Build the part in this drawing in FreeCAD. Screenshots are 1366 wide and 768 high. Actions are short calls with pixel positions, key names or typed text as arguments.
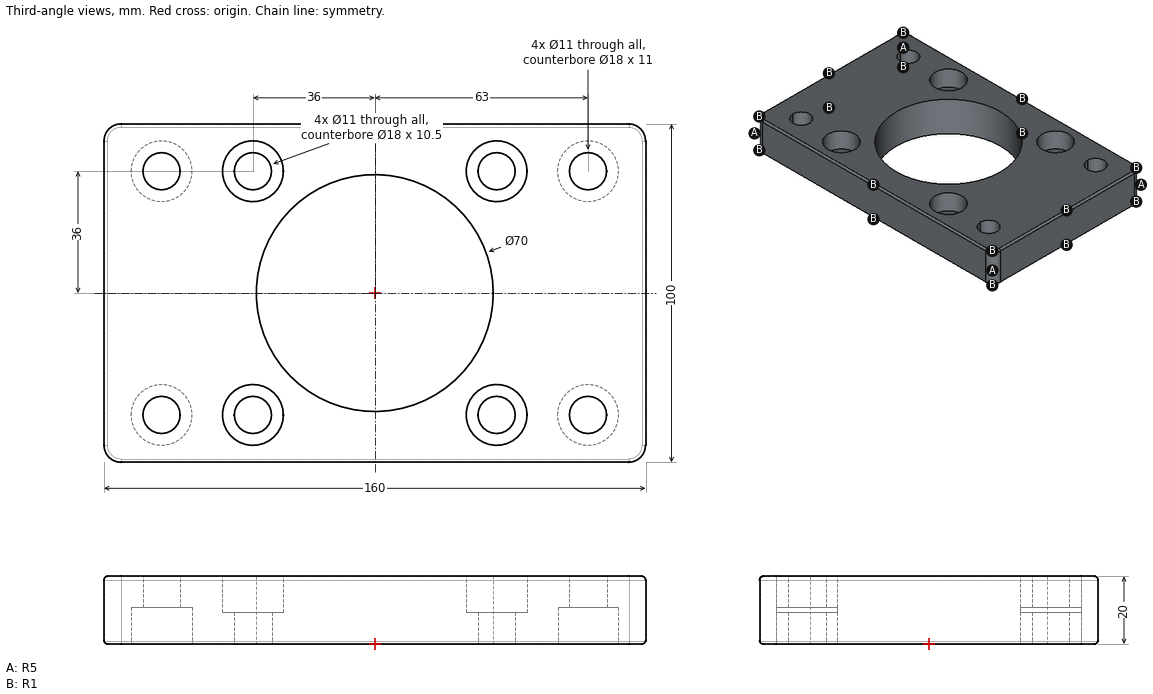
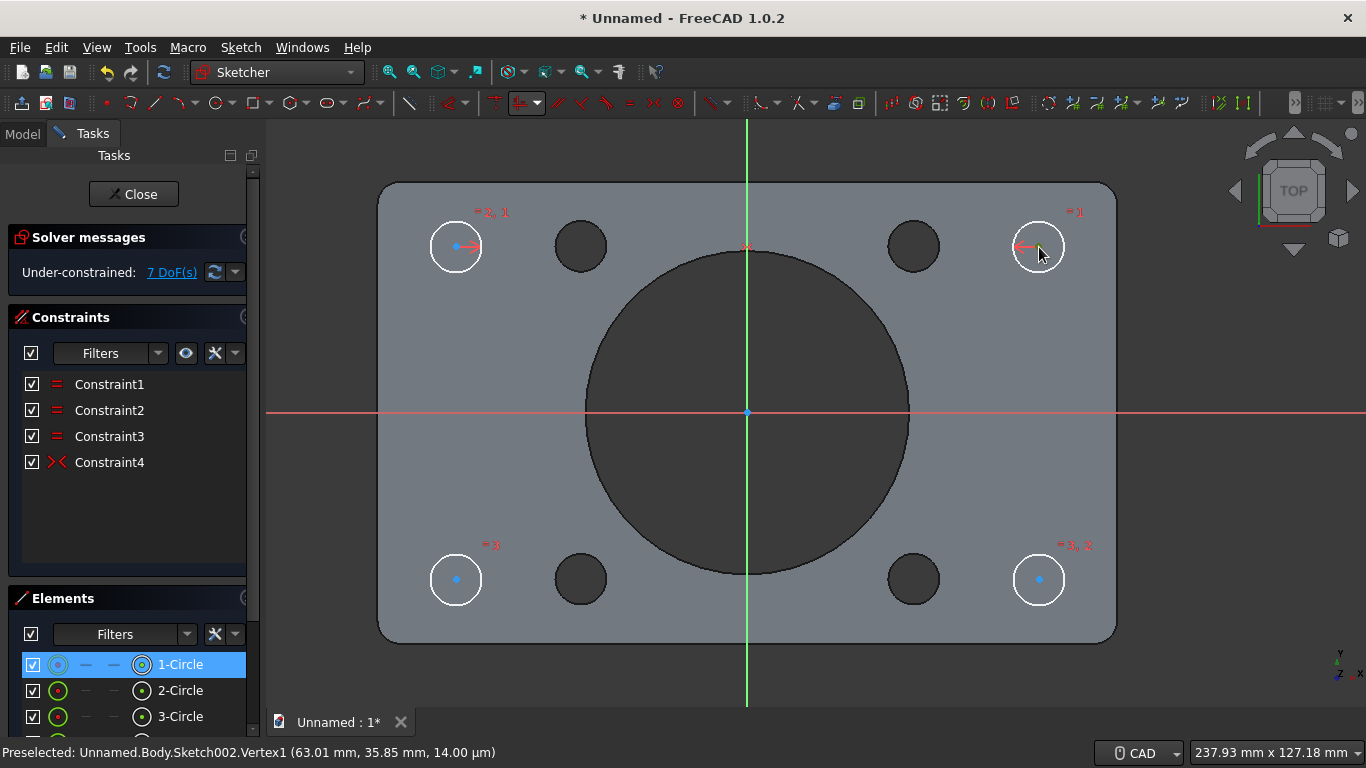
click(1039, 580)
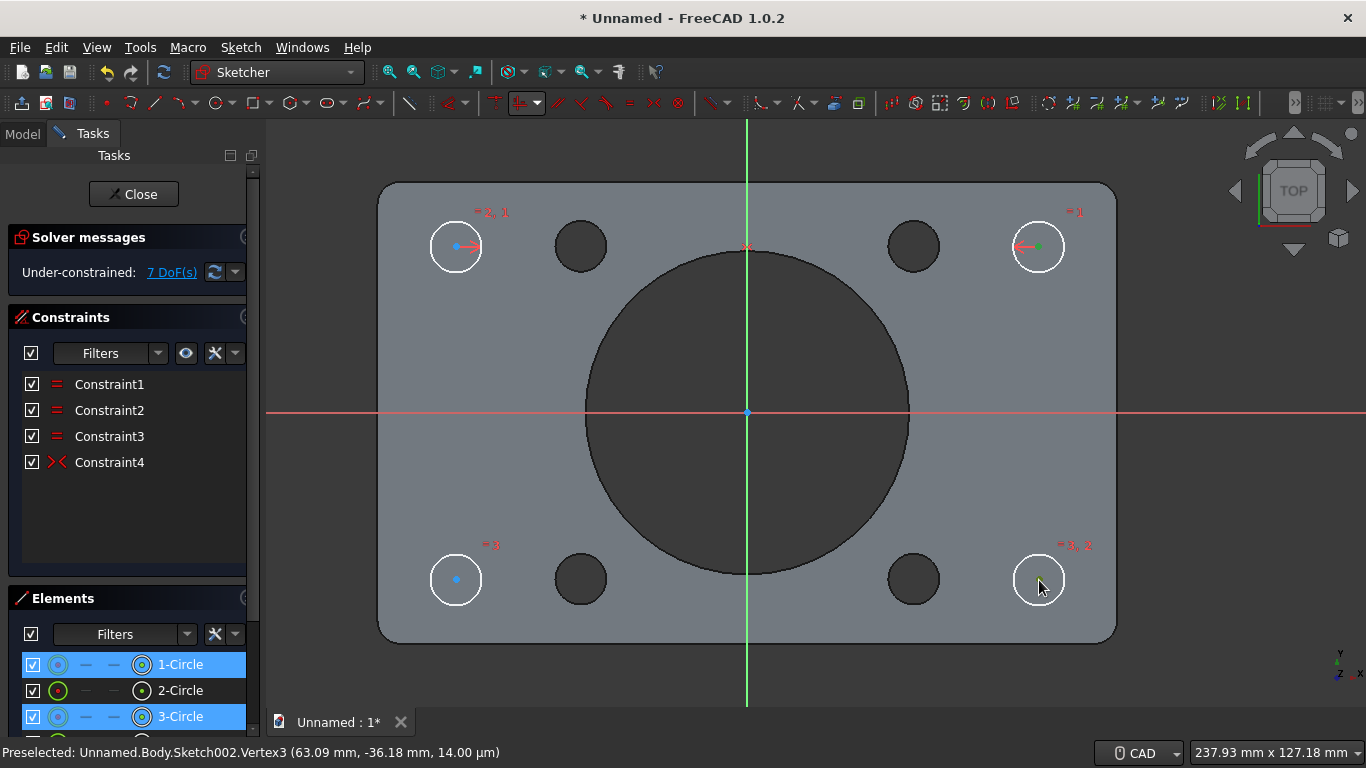
click(359, 413)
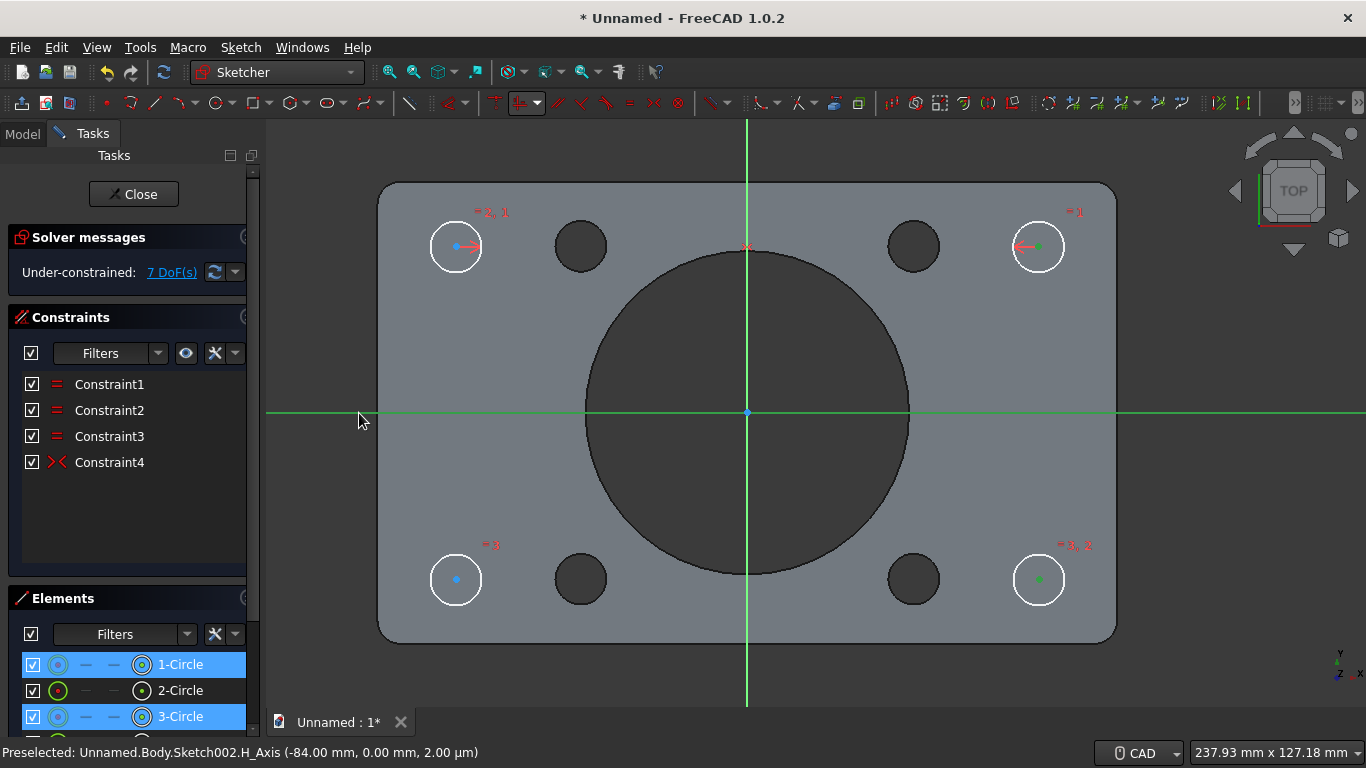
click(654, 104)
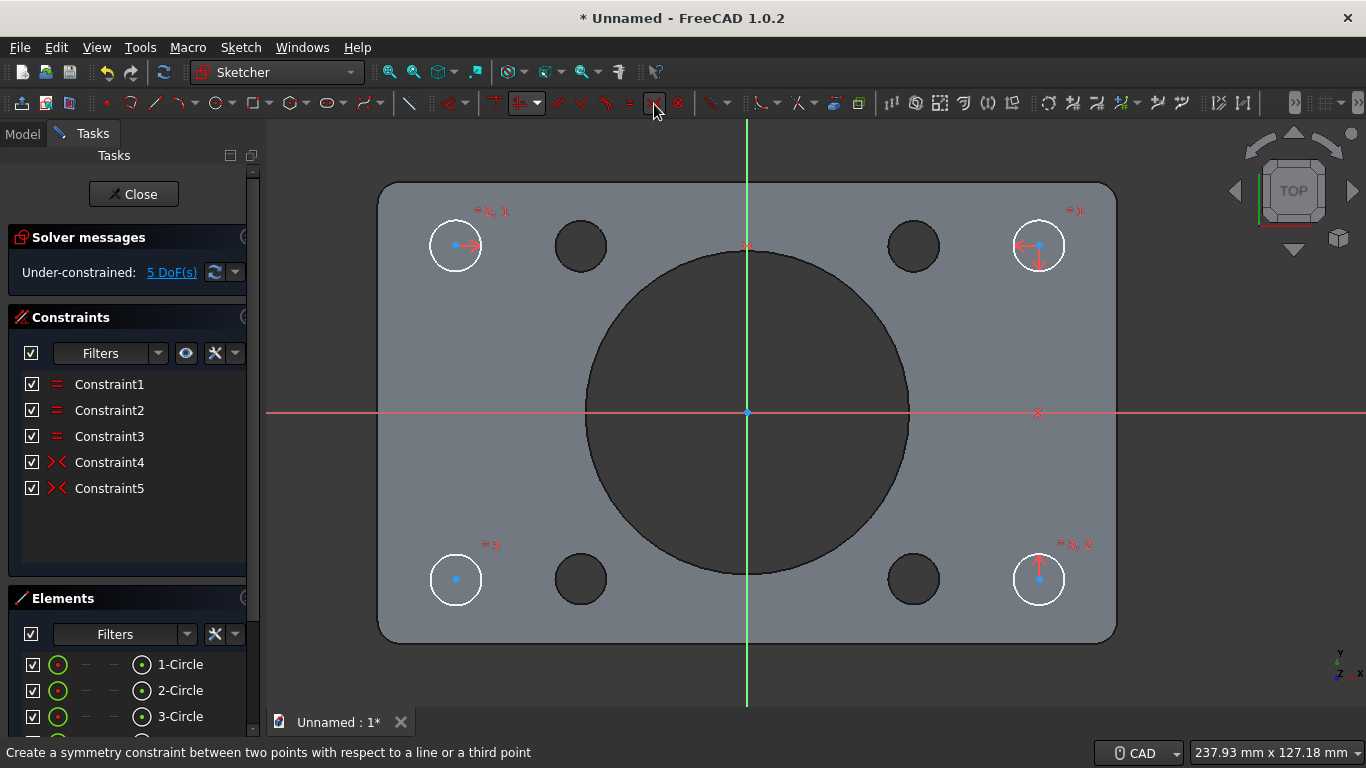
click(456, 246)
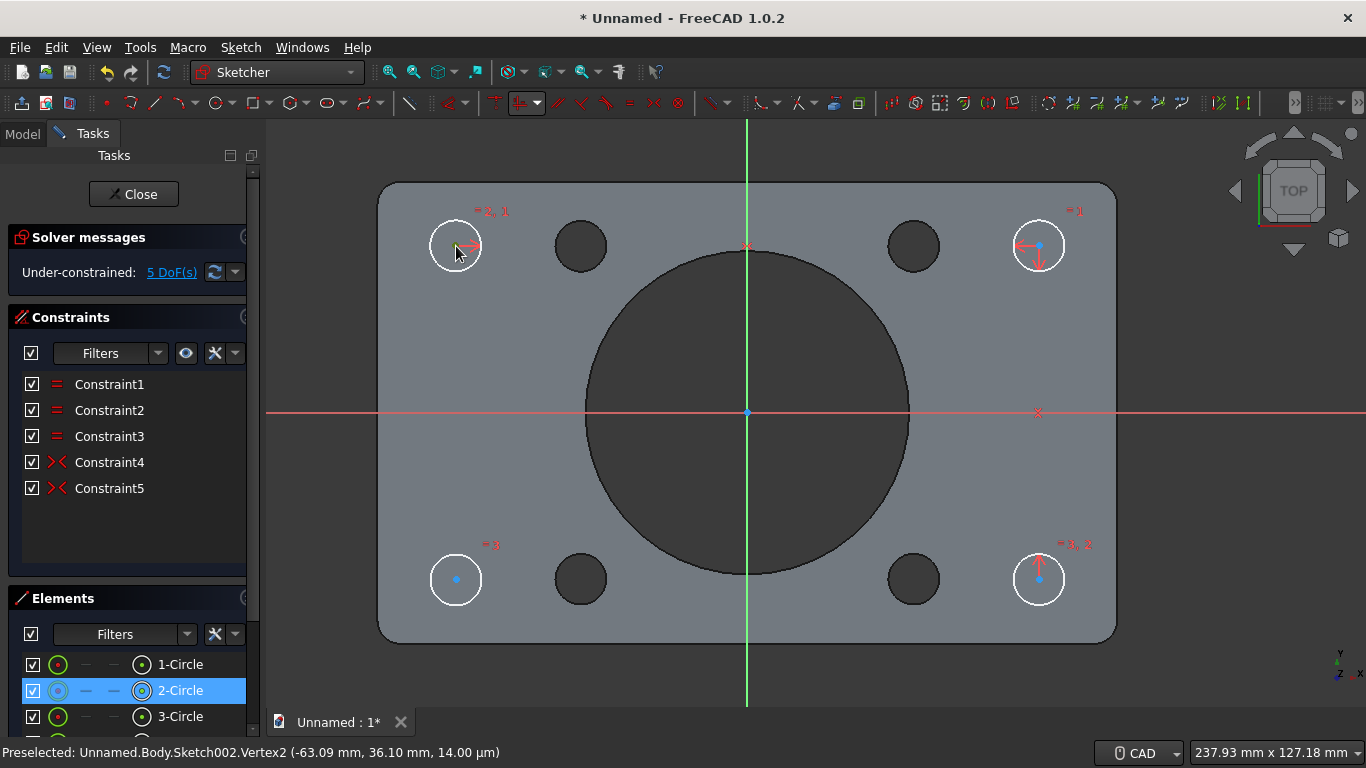
click(456, 580)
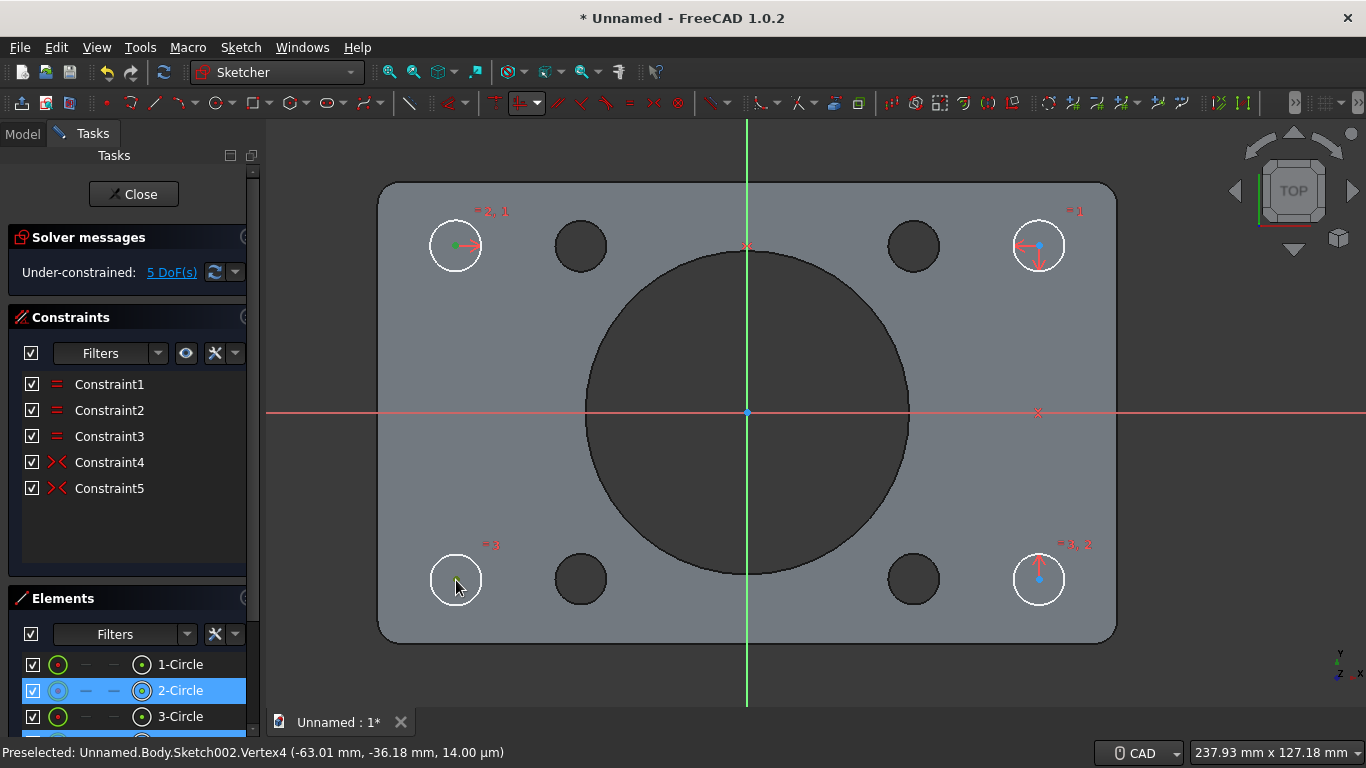
click(359, 413)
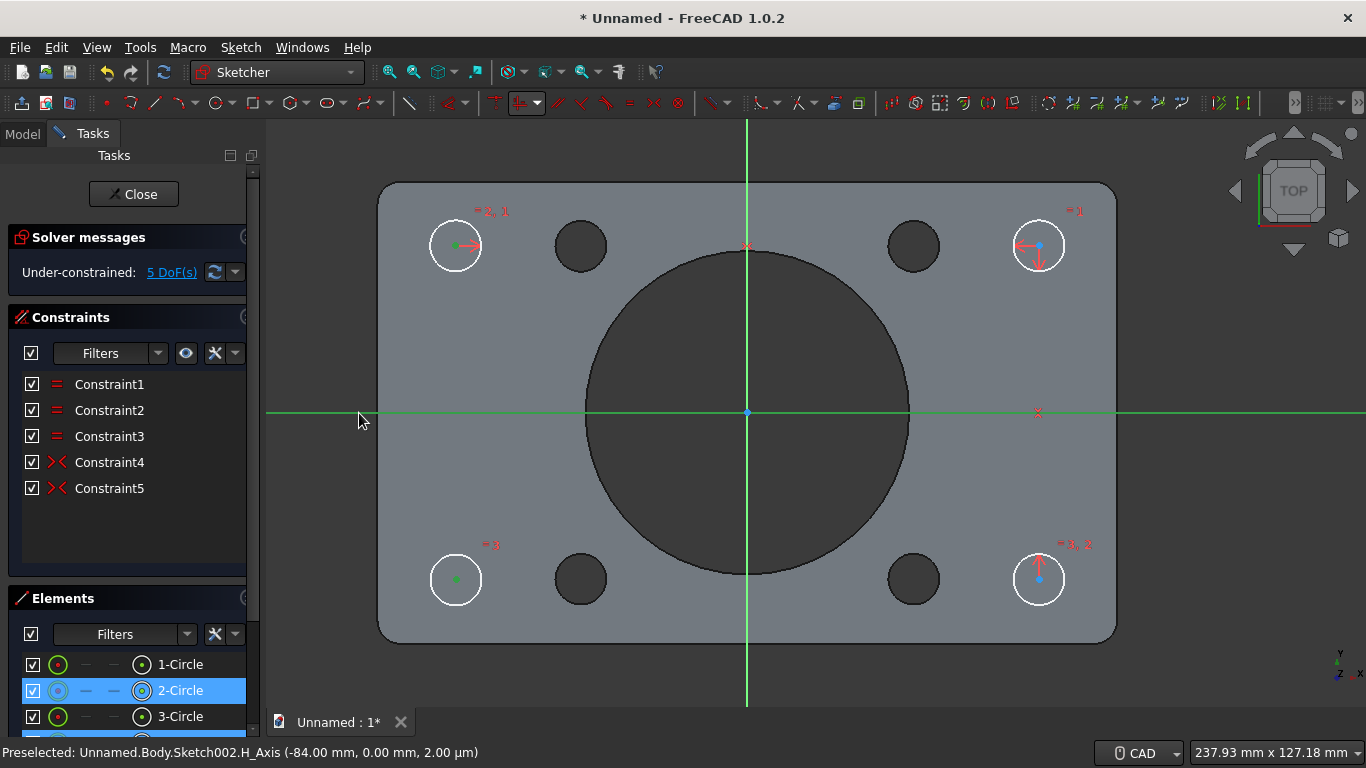
click(654, 104)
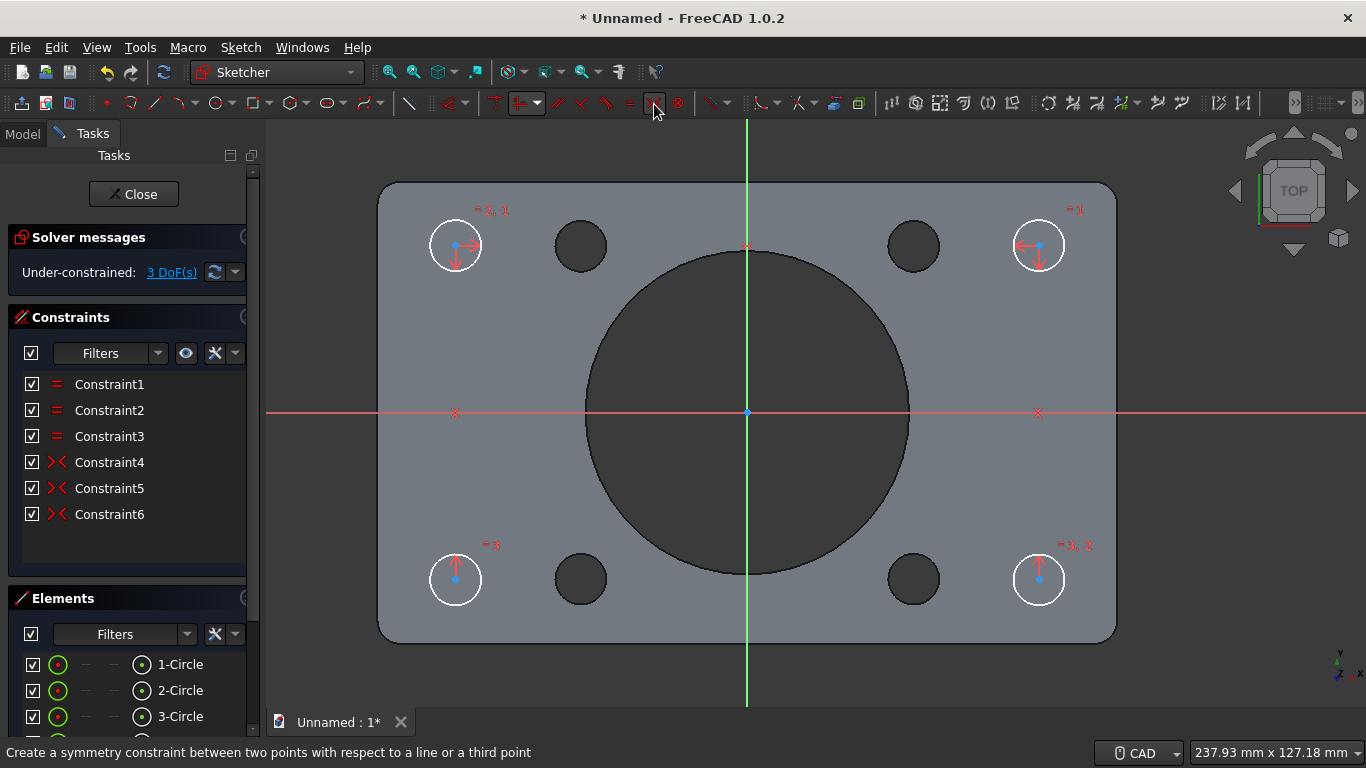
click(448, 104)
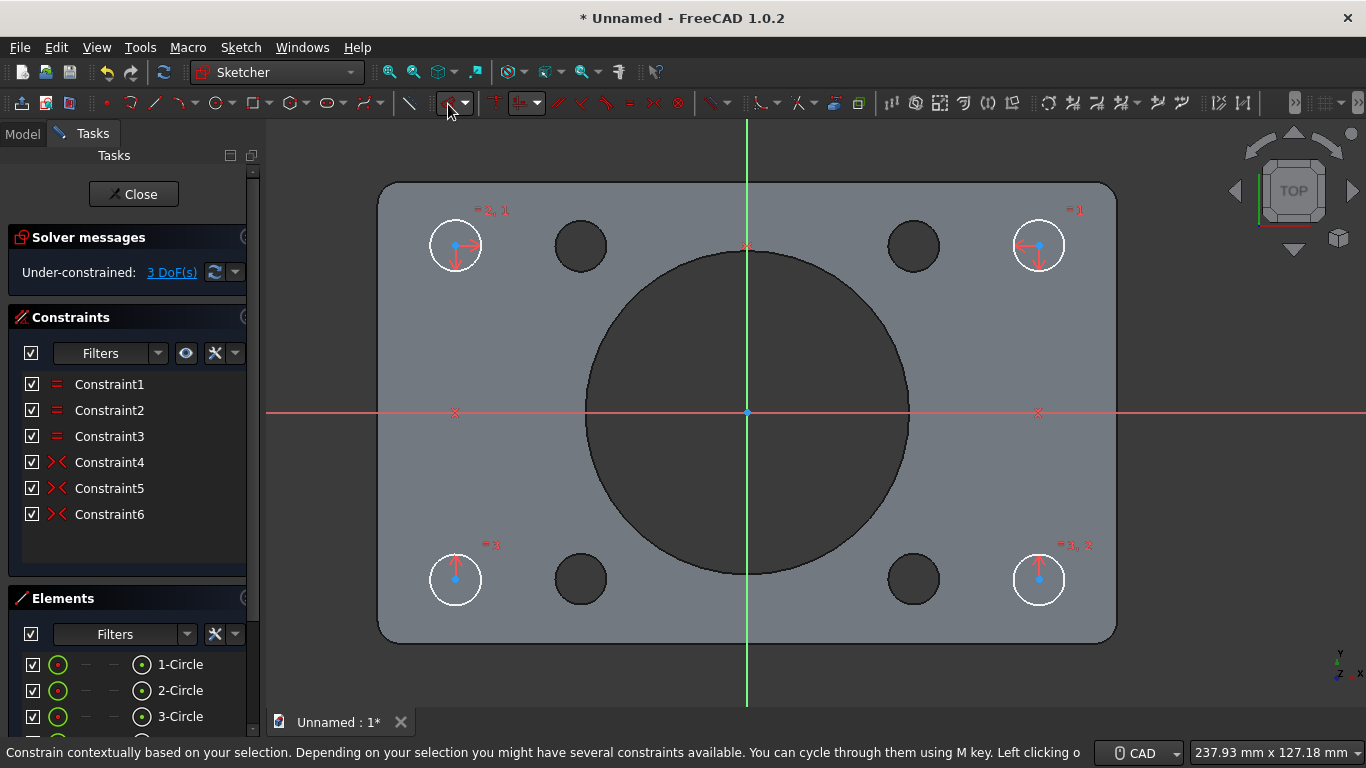
click(1057, 228)
click(1080, 206)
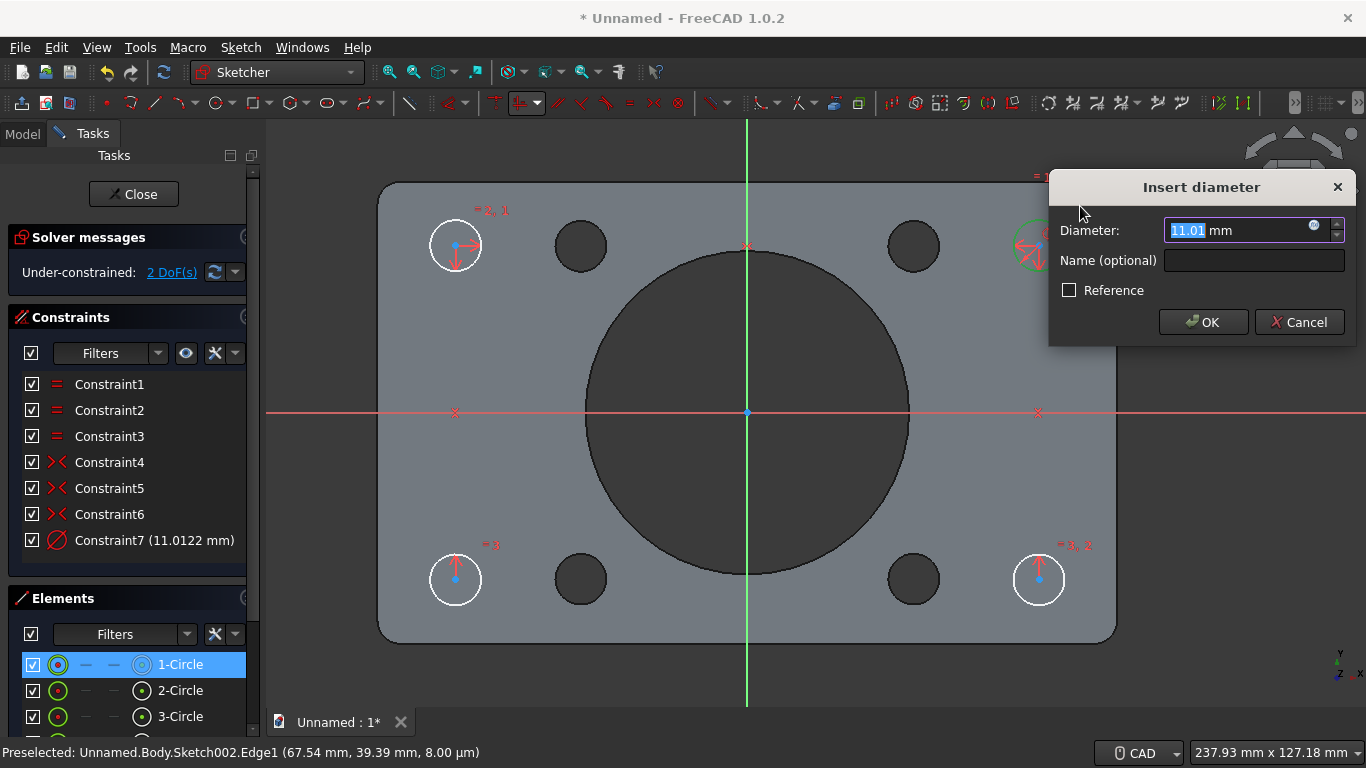
text(11)
key(Return)